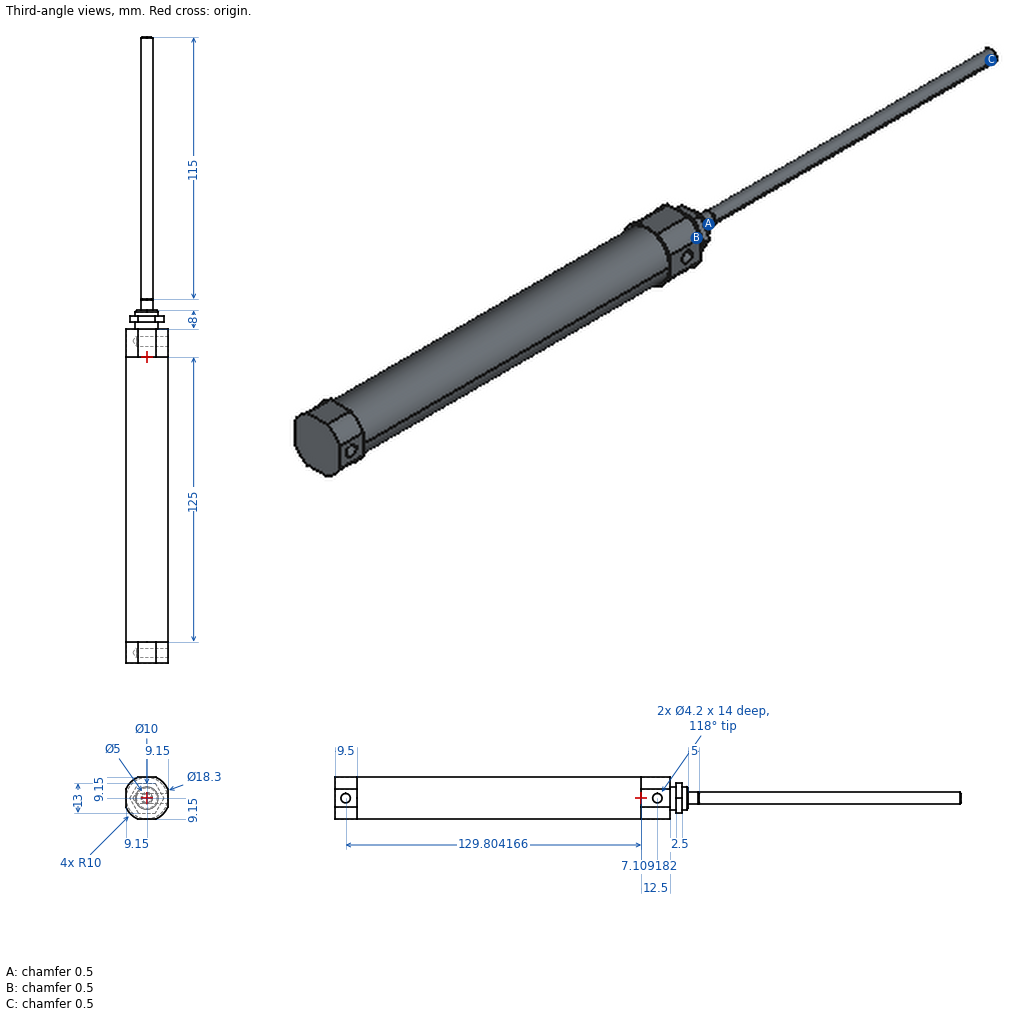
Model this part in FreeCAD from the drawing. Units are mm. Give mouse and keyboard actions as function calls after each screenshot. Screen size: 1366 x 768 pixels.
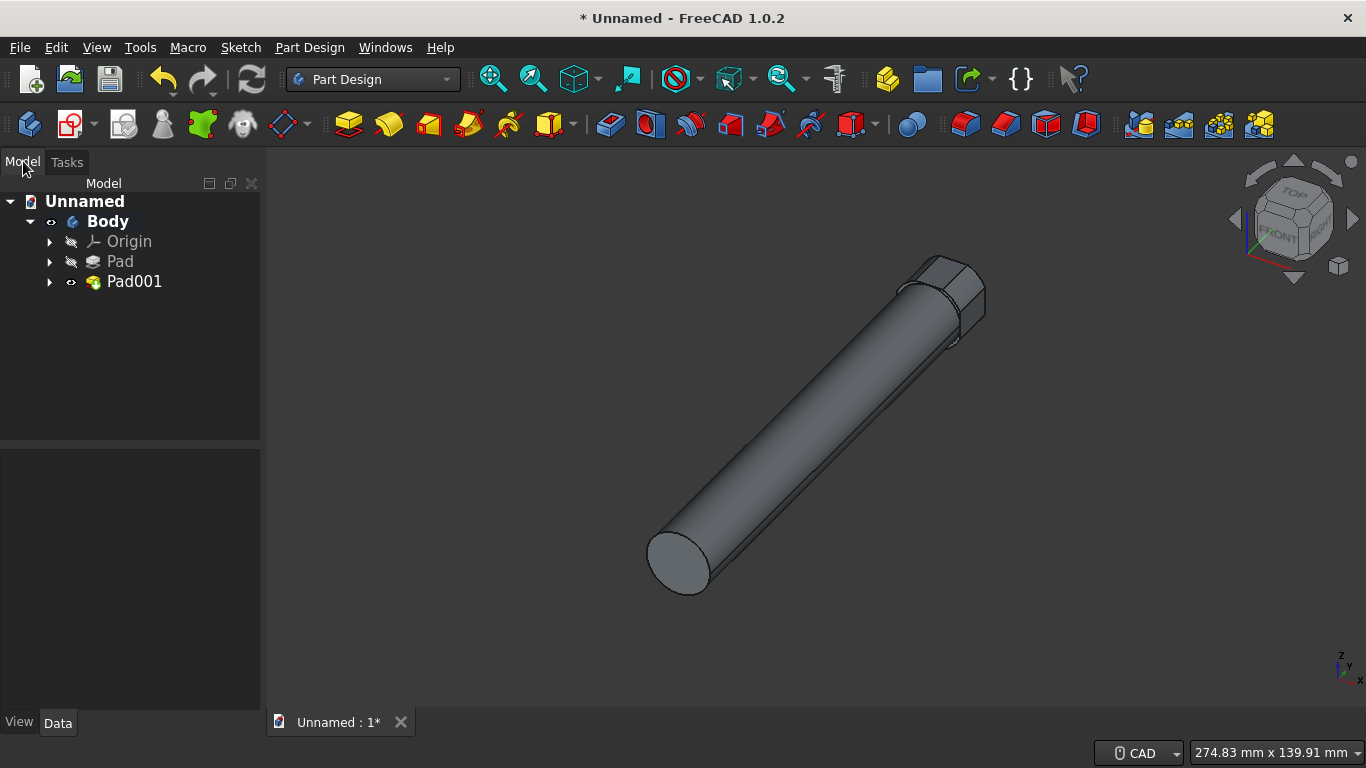
click(50, 242)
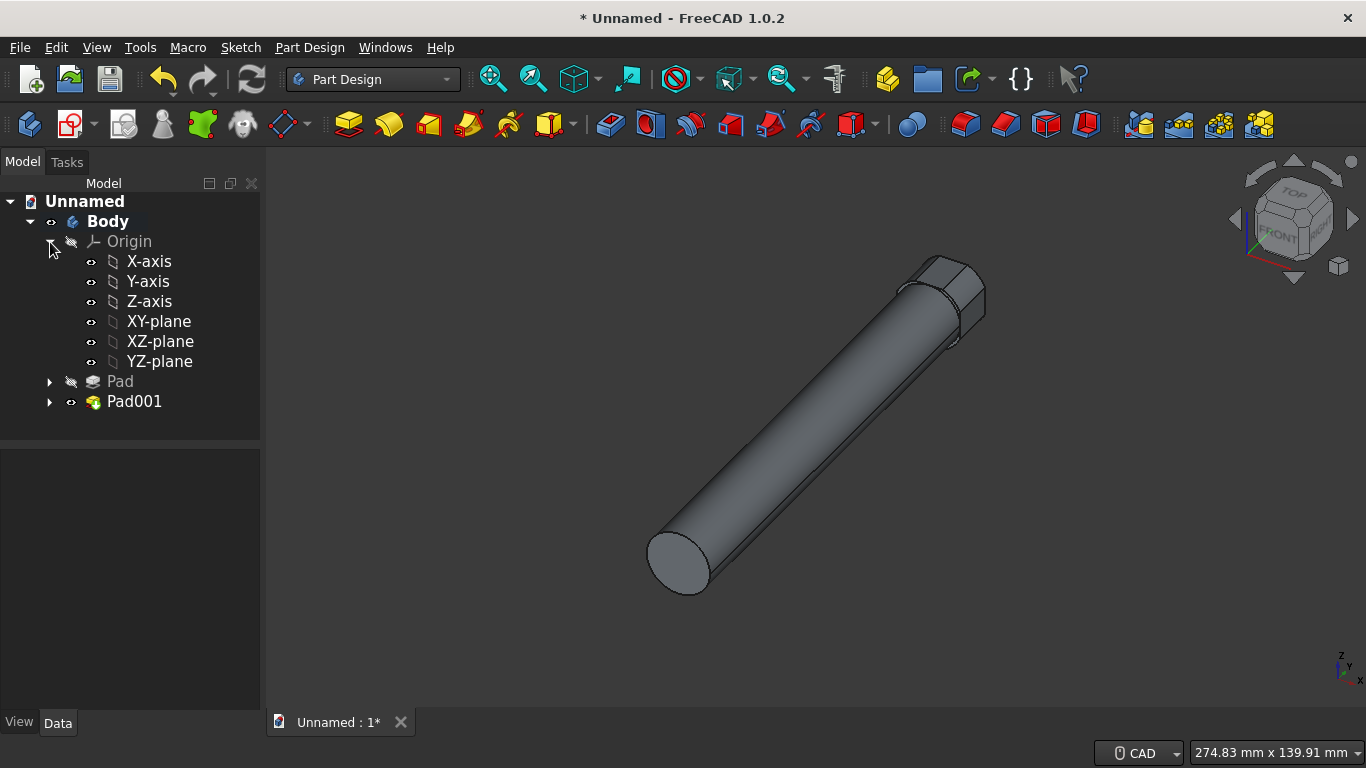
click(136, 342)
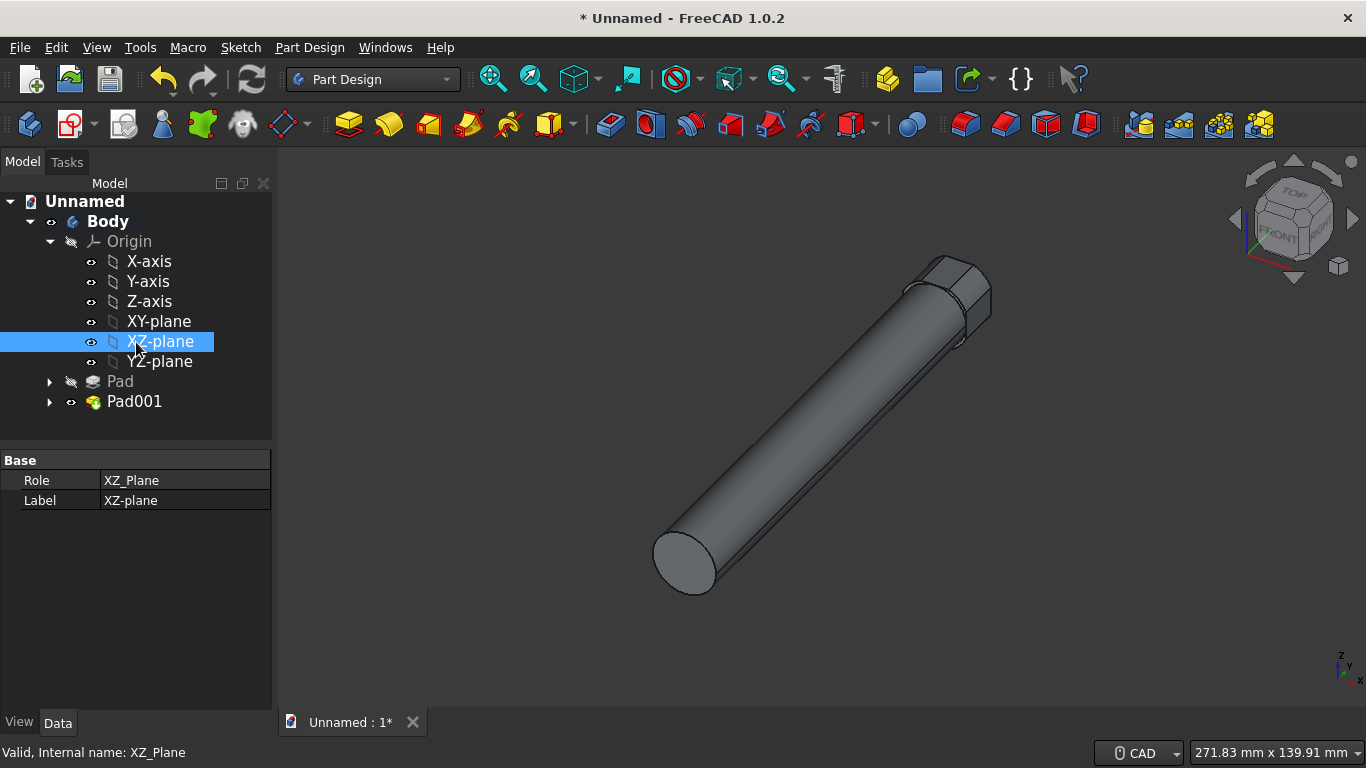
click(284, 124)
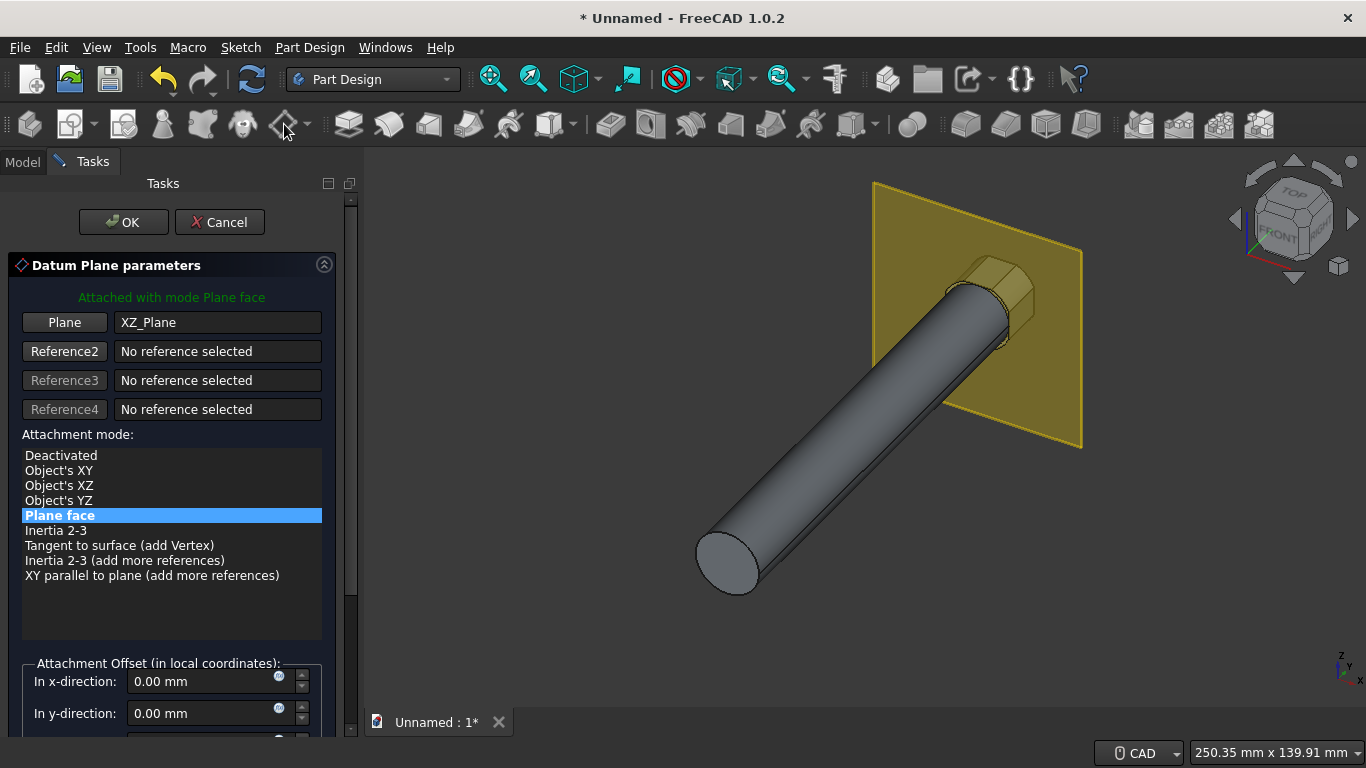
scroll(351, 464, down, 2)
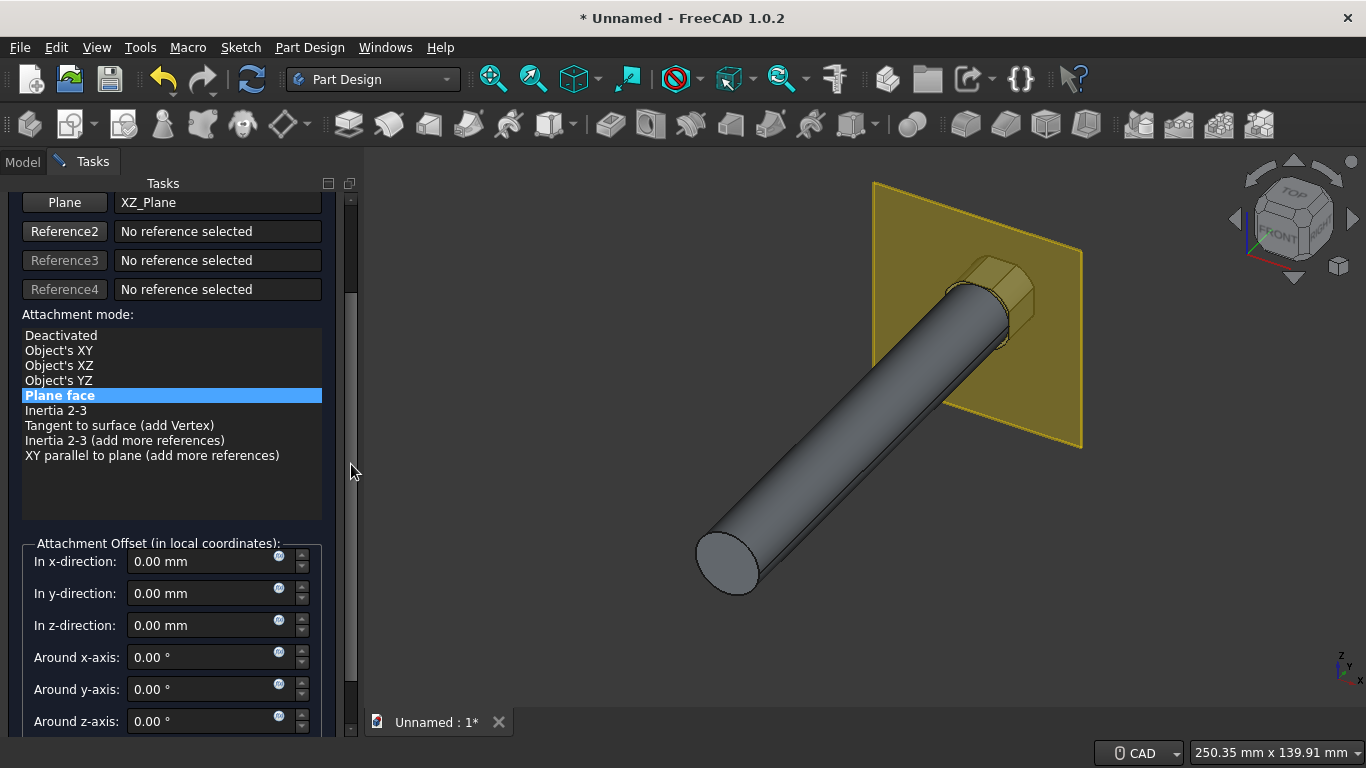
triple_click(210, 625)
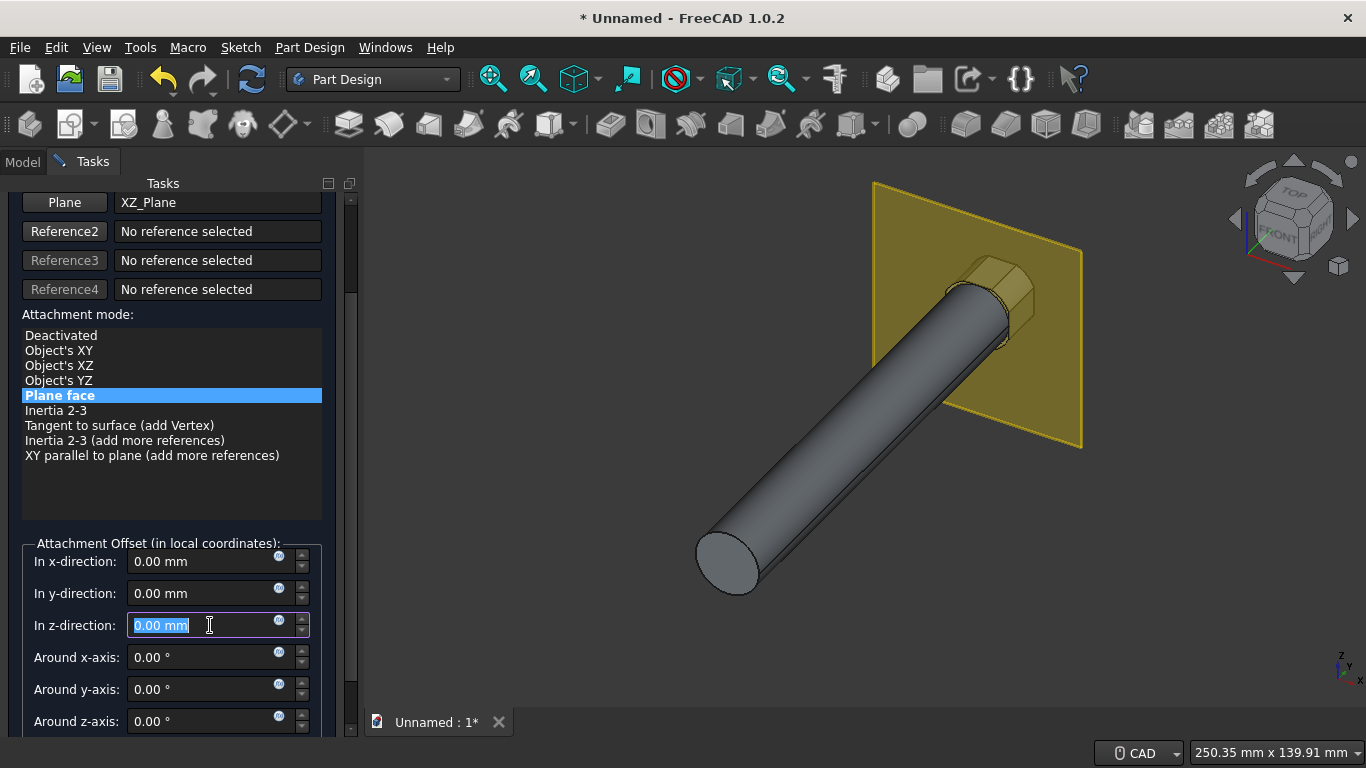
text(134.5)
key(Tab)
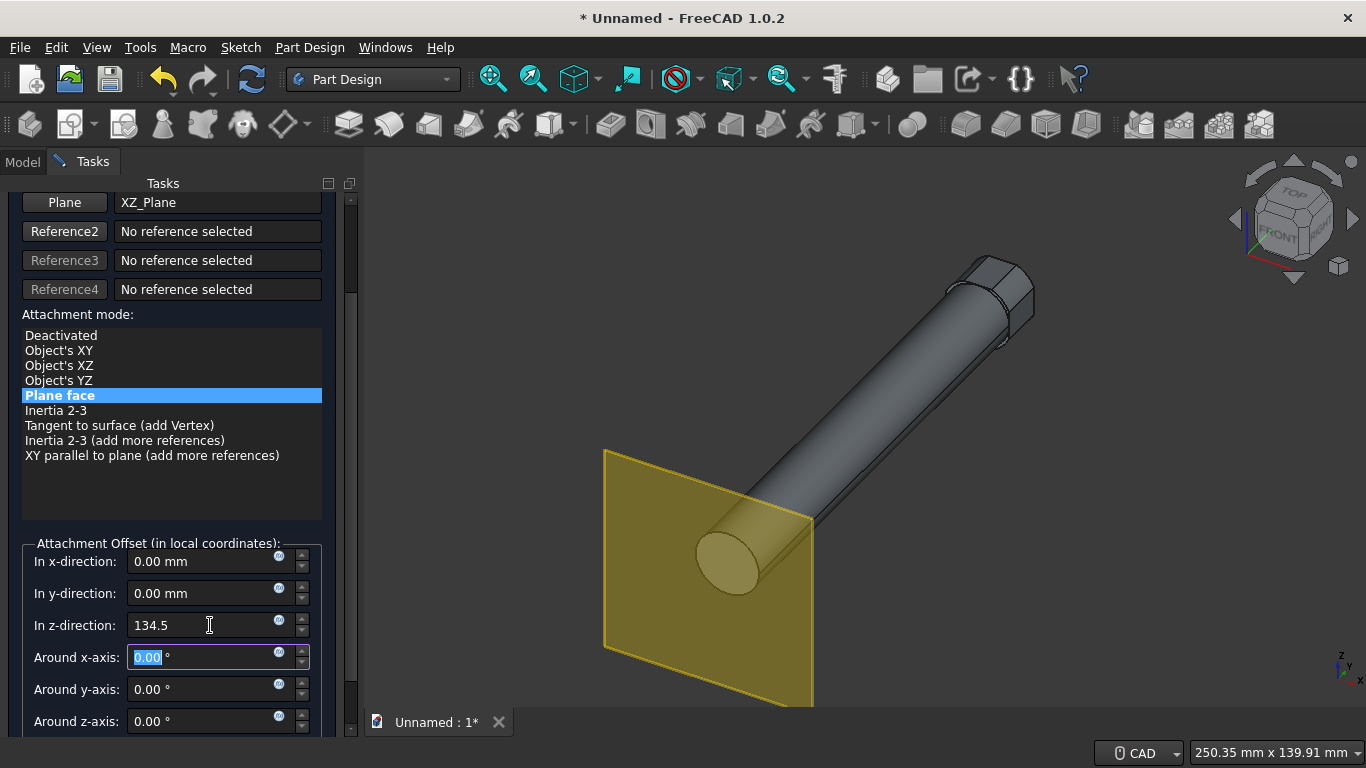
scroll(351, 464, up, 3)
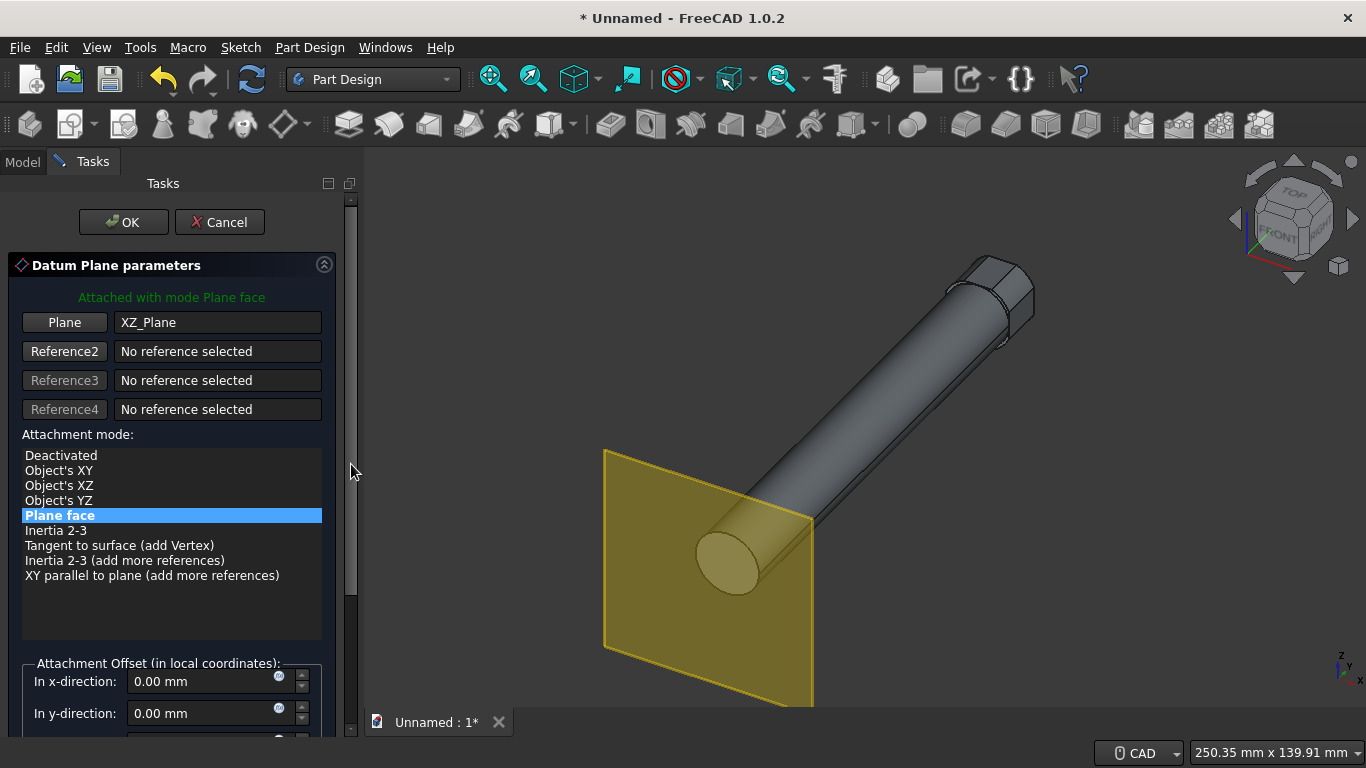
click(124, 222)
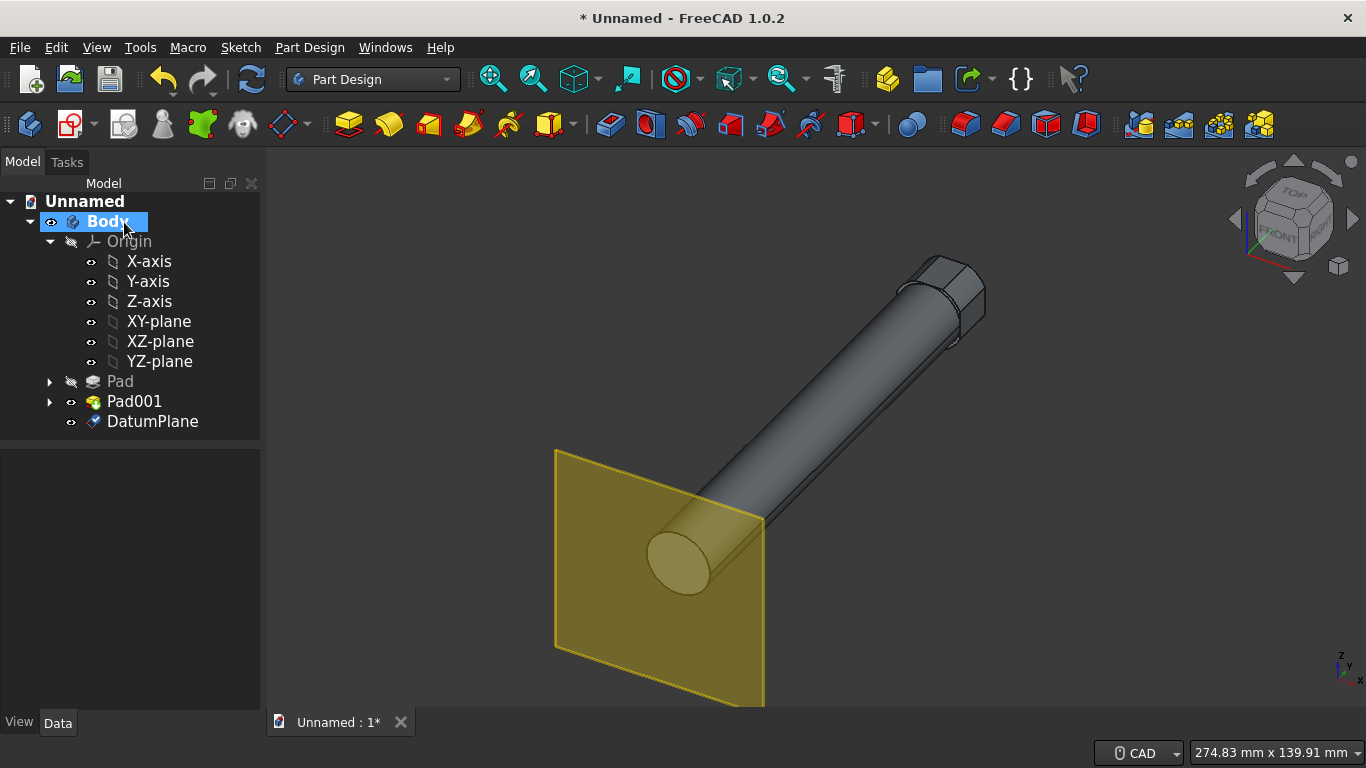
click(116, 422)